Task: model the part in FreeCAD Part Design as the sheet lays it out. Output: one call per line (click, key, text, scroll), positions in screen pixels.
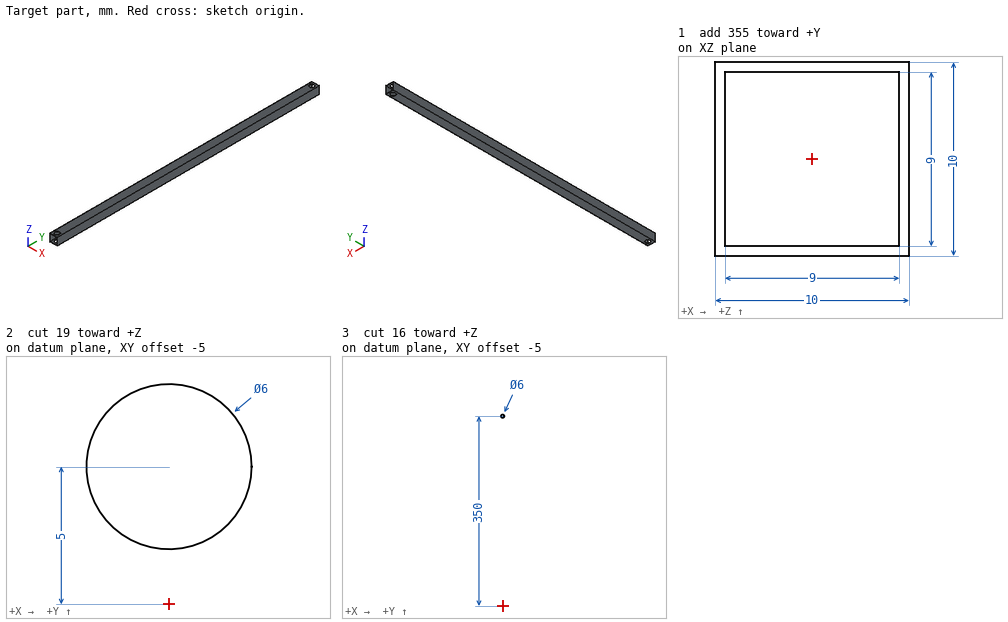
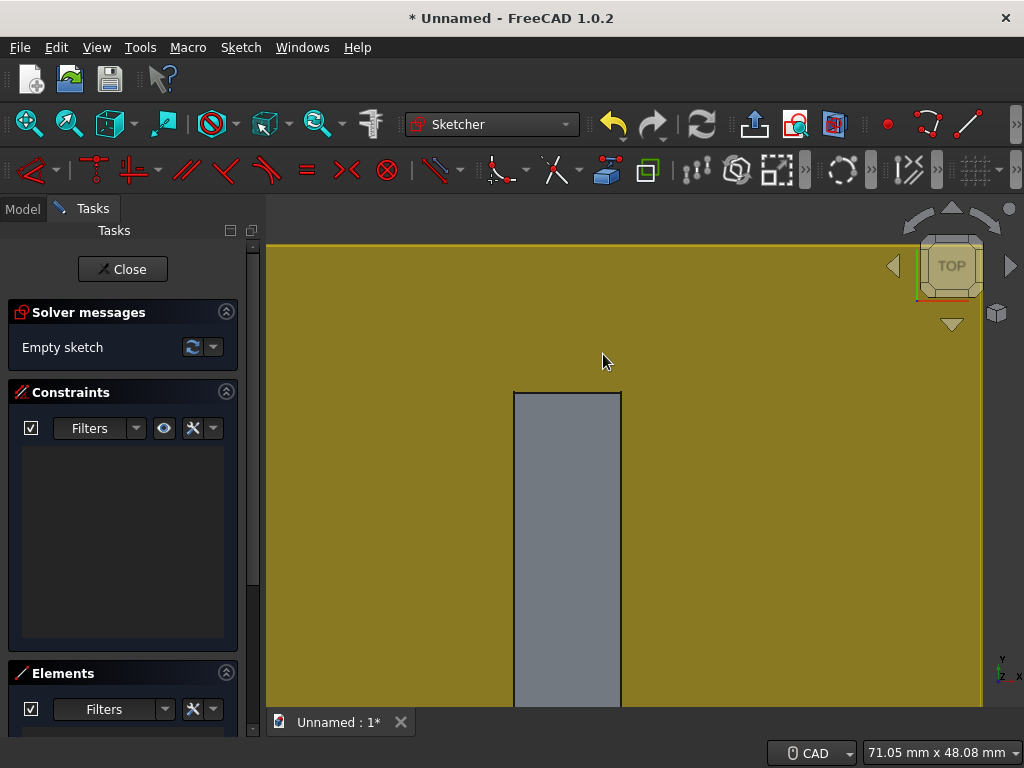
scroll(565, 445, up, 8)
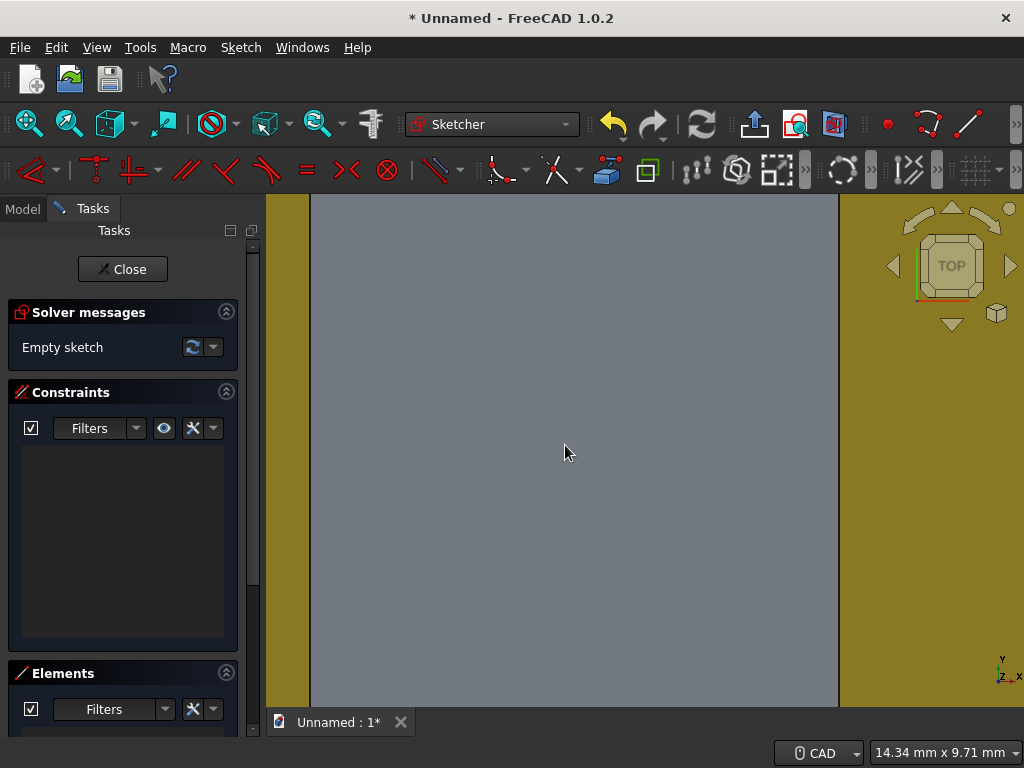
key(g)
key(c)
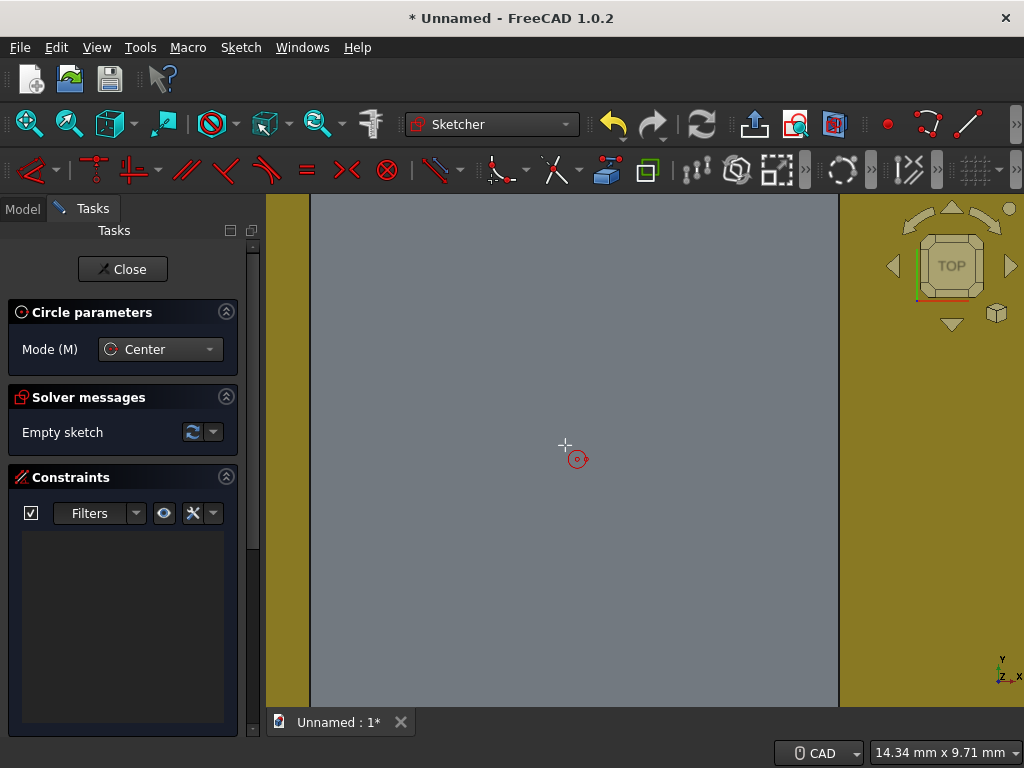
click(575, 447)
move(687, 335)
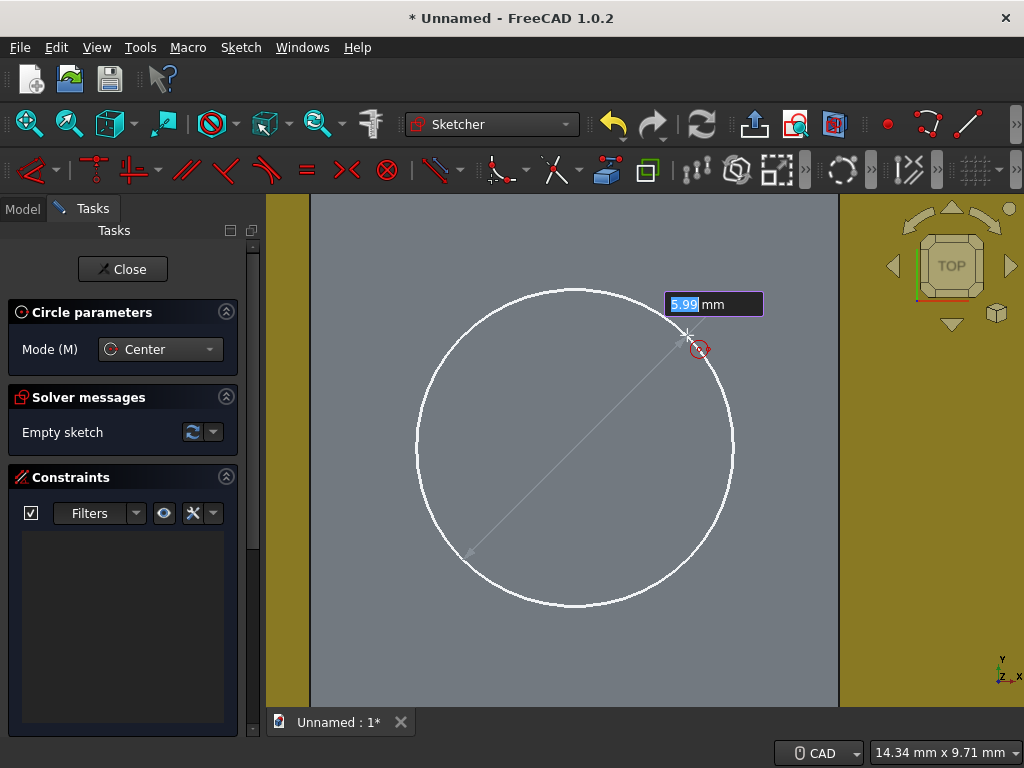
text(6)
key(Return)
key(Escape)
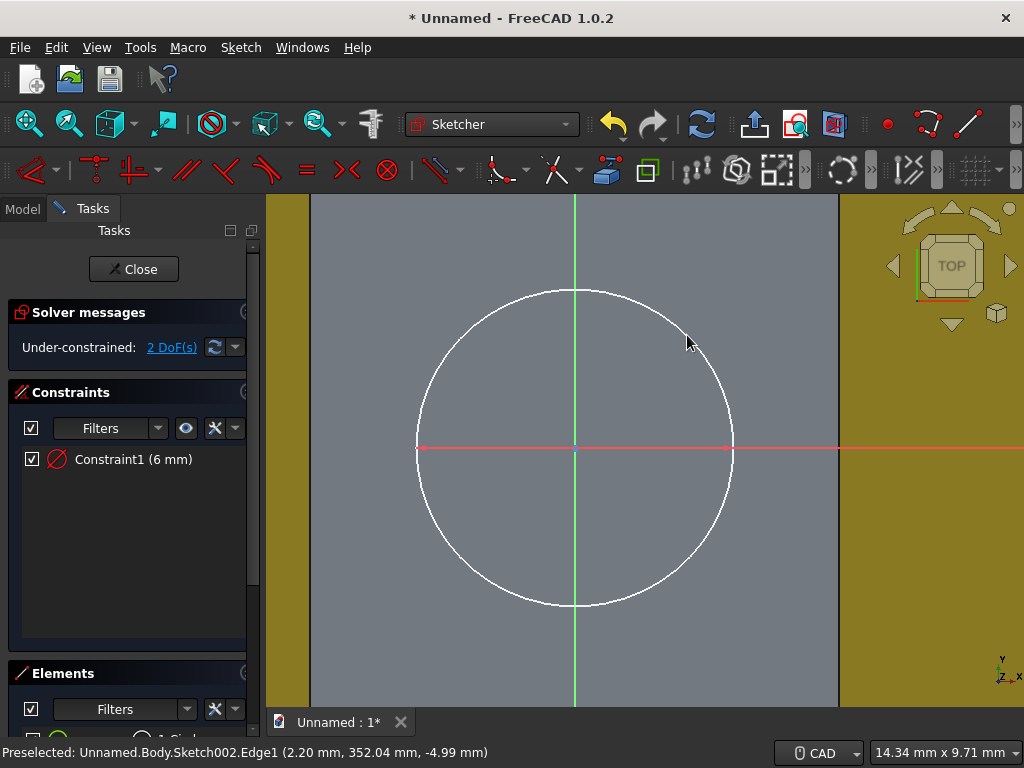
click(575, 448)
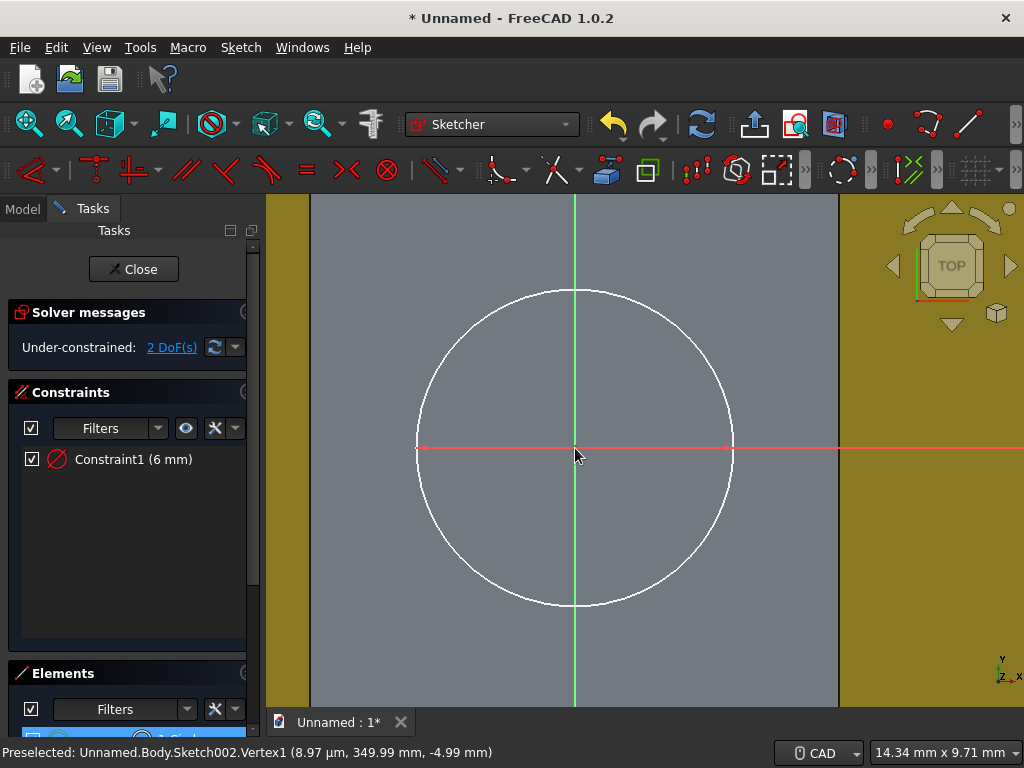
click(575, 646)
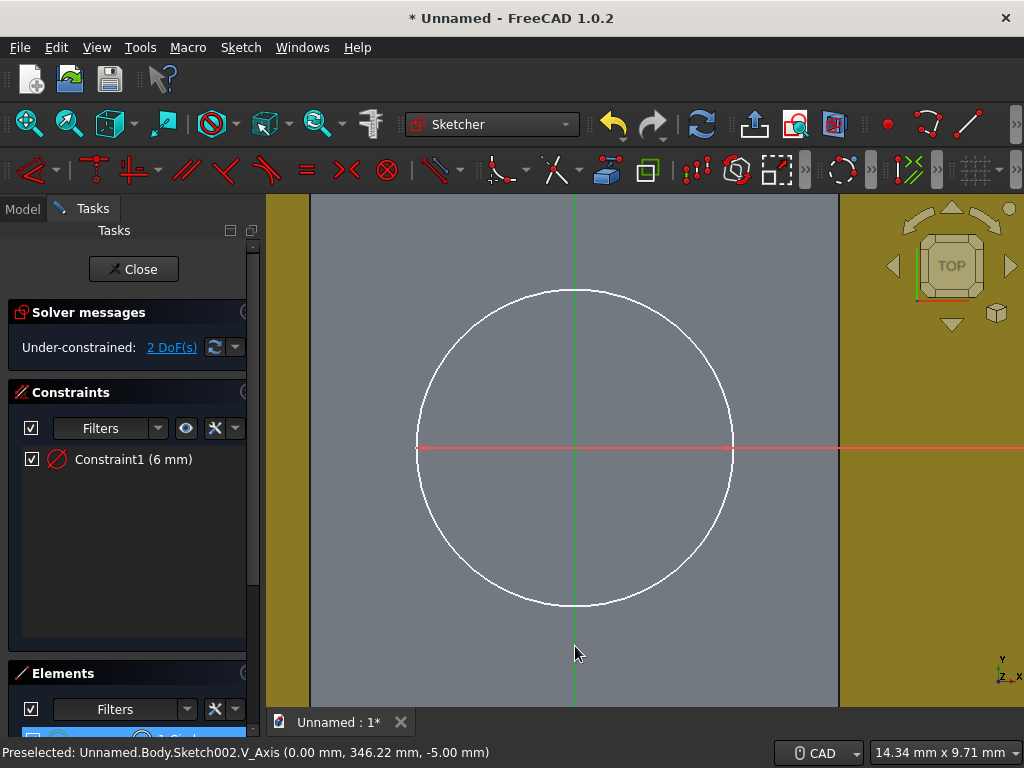
click(94, 170)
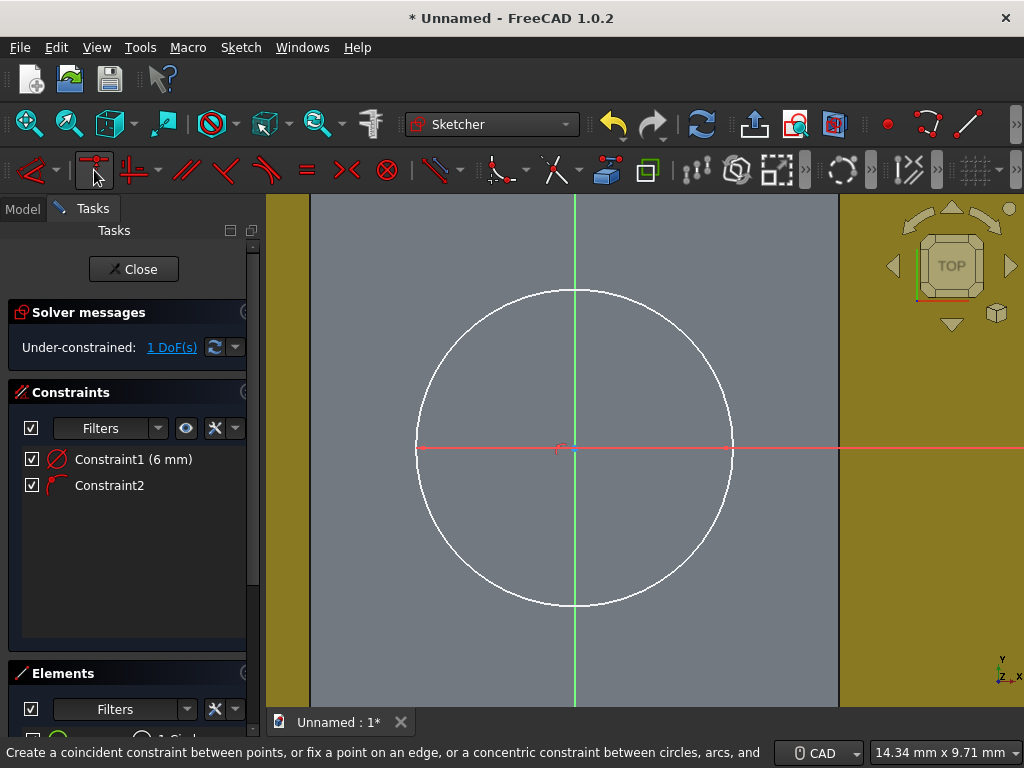
click(32, 170)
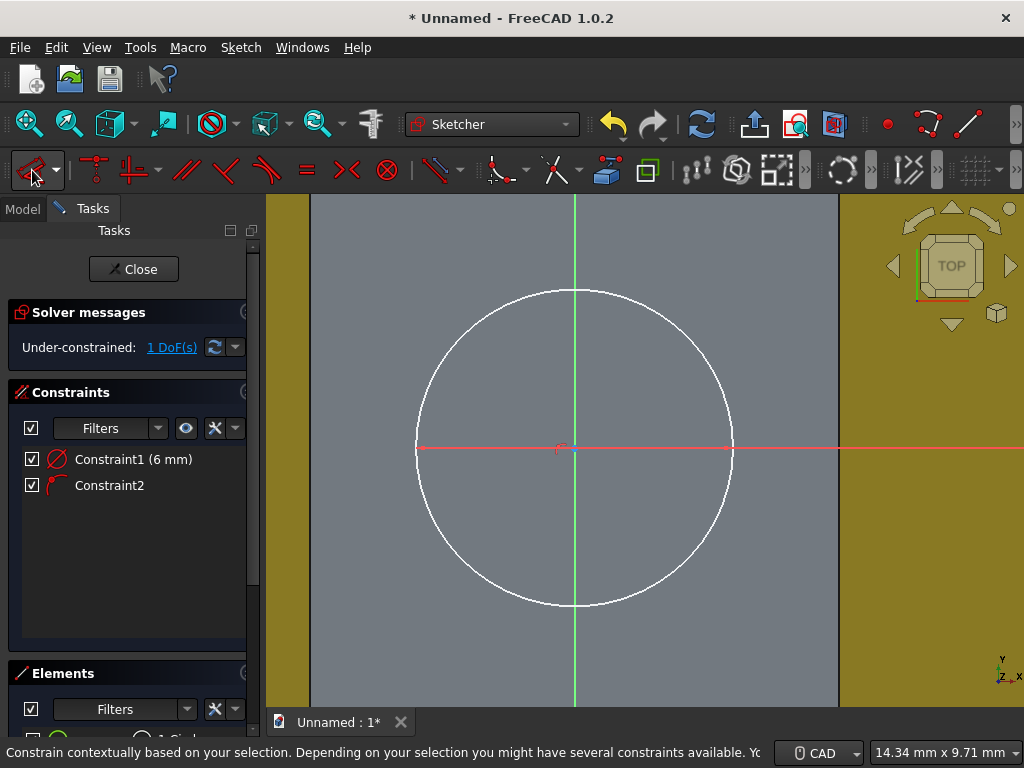
click(575, 448)
click(609, 564)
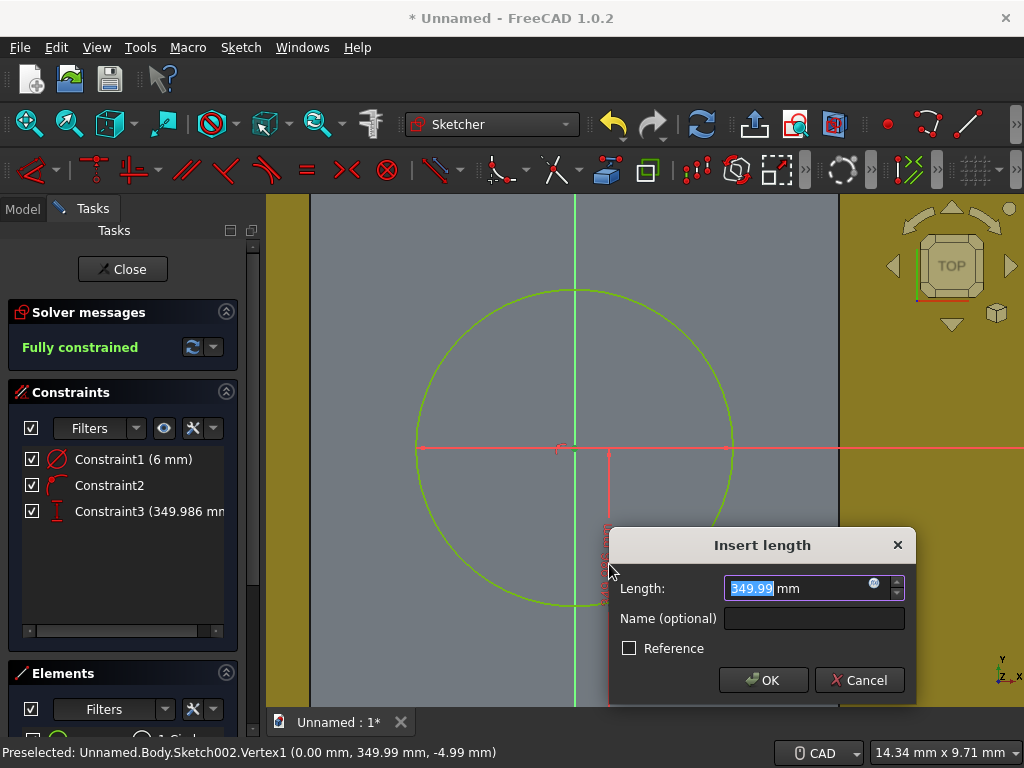
text(350)
key(Return)
key(Escape)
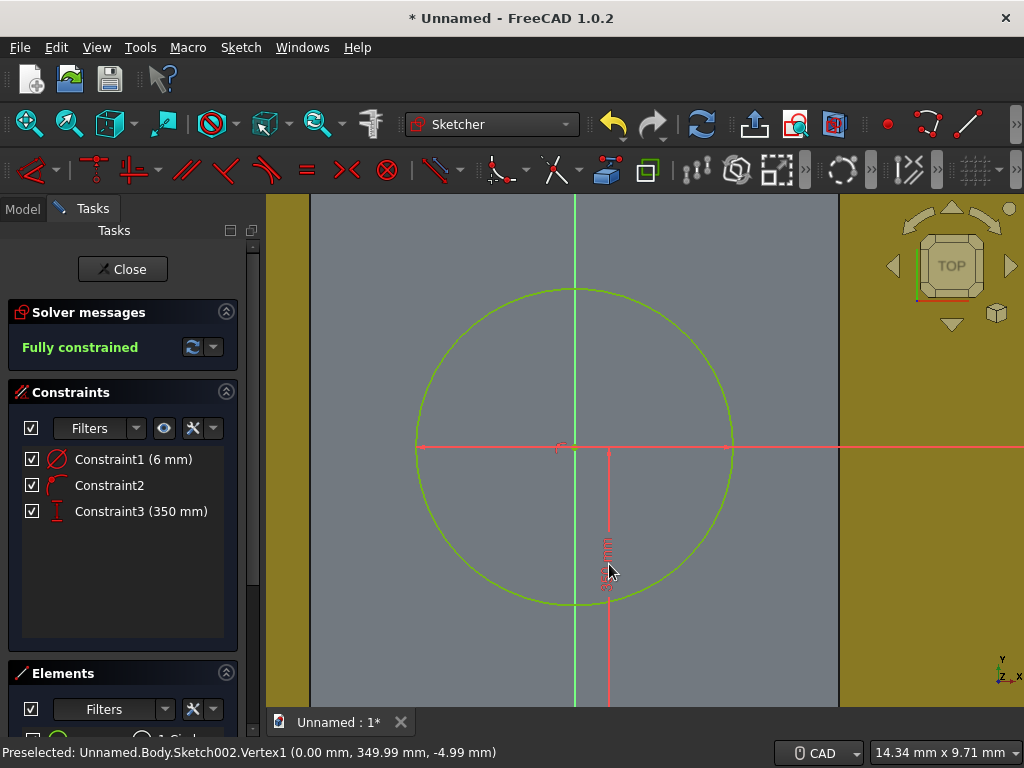
click(123, 269)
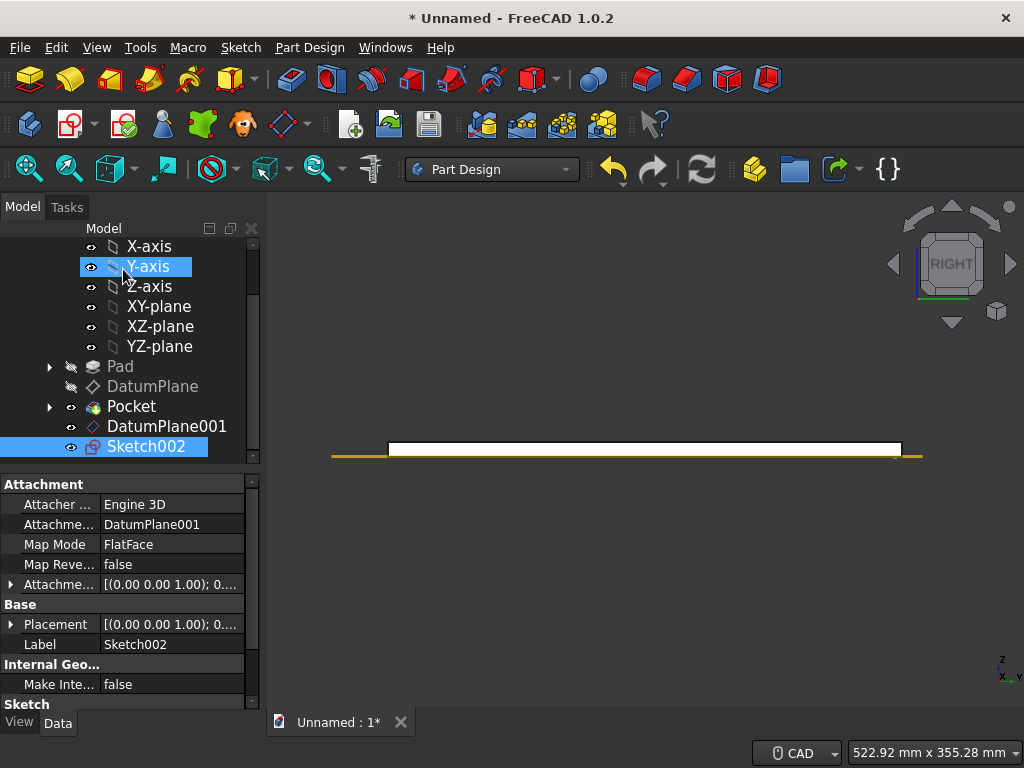
click(292, 80)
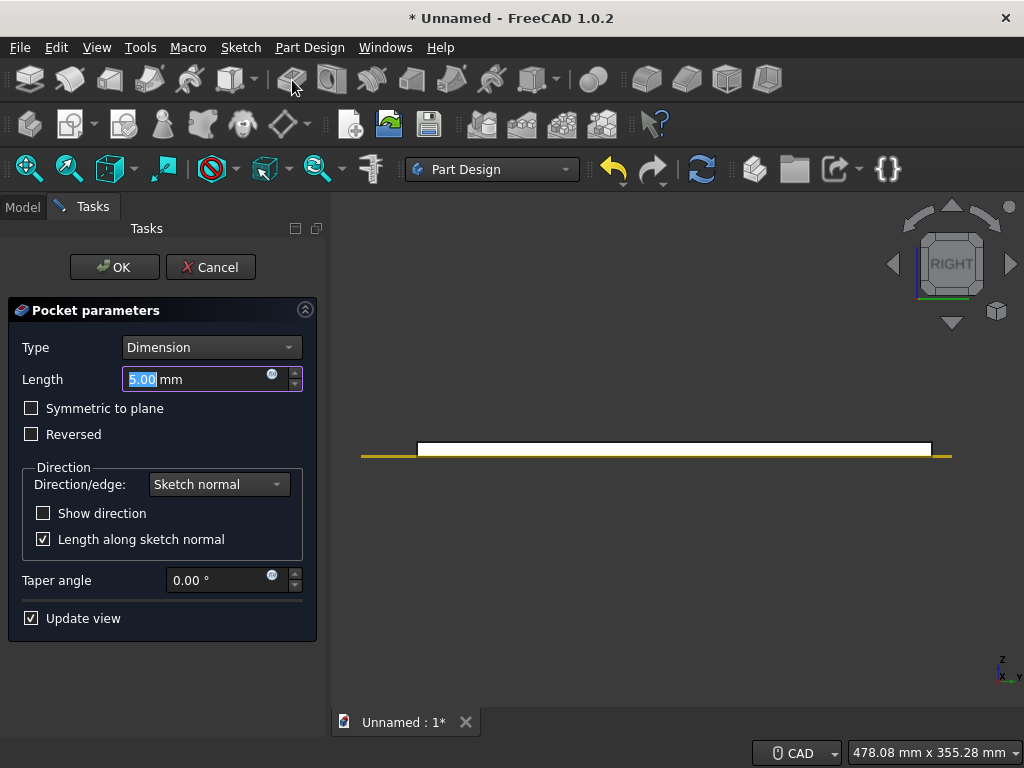
text(16)
key(Tab)